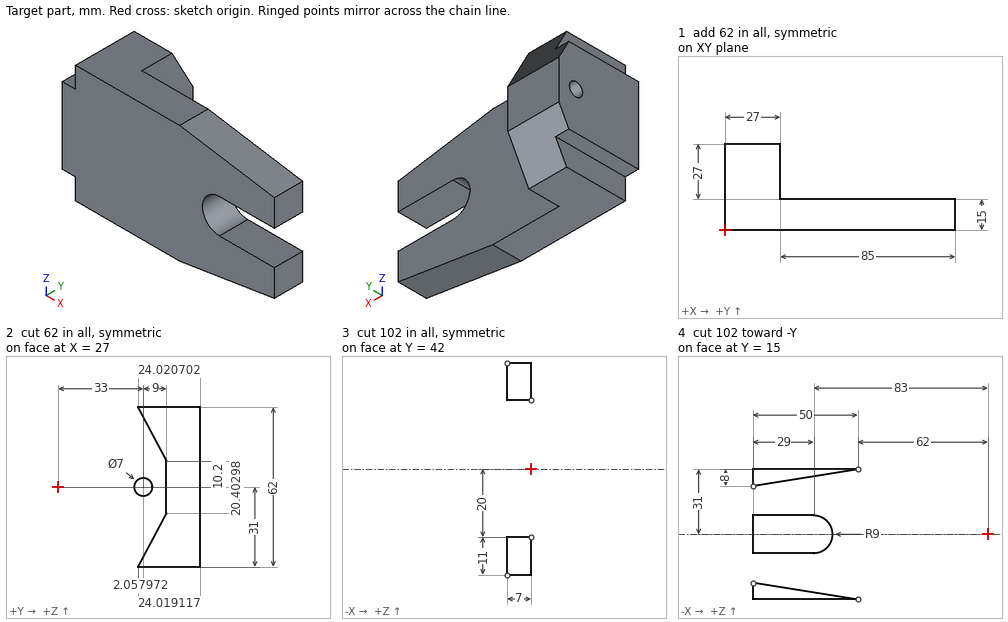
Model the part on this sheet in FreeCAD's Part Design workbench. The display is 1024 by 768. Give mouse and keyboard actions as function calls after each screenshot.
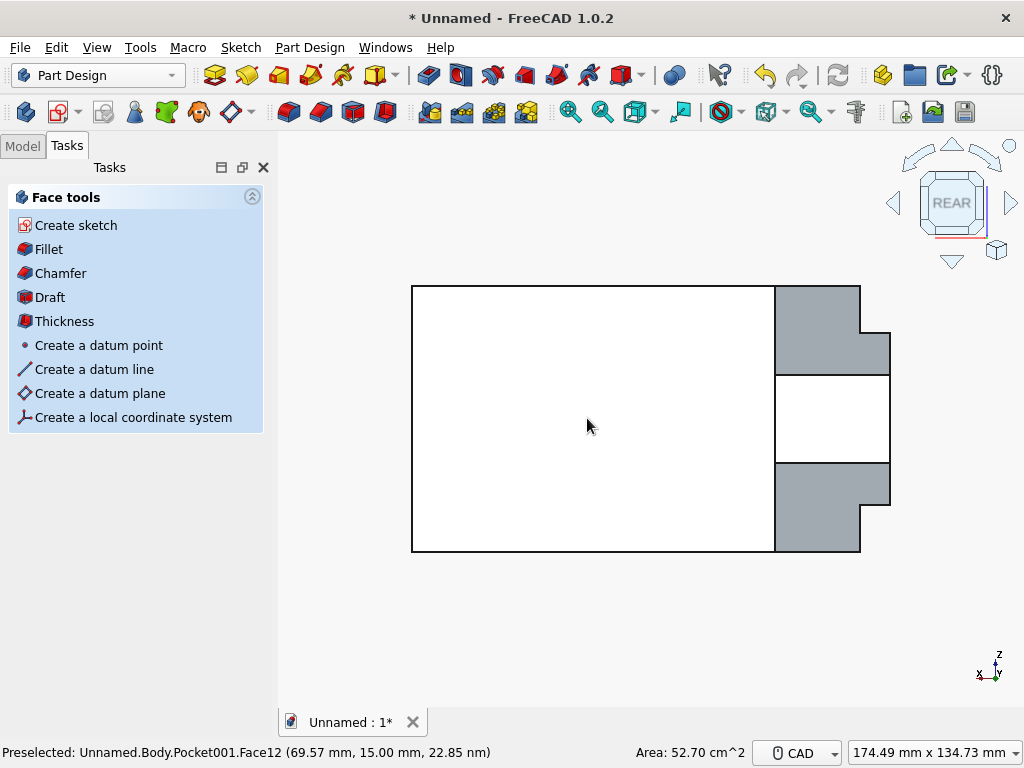
click(58, 112)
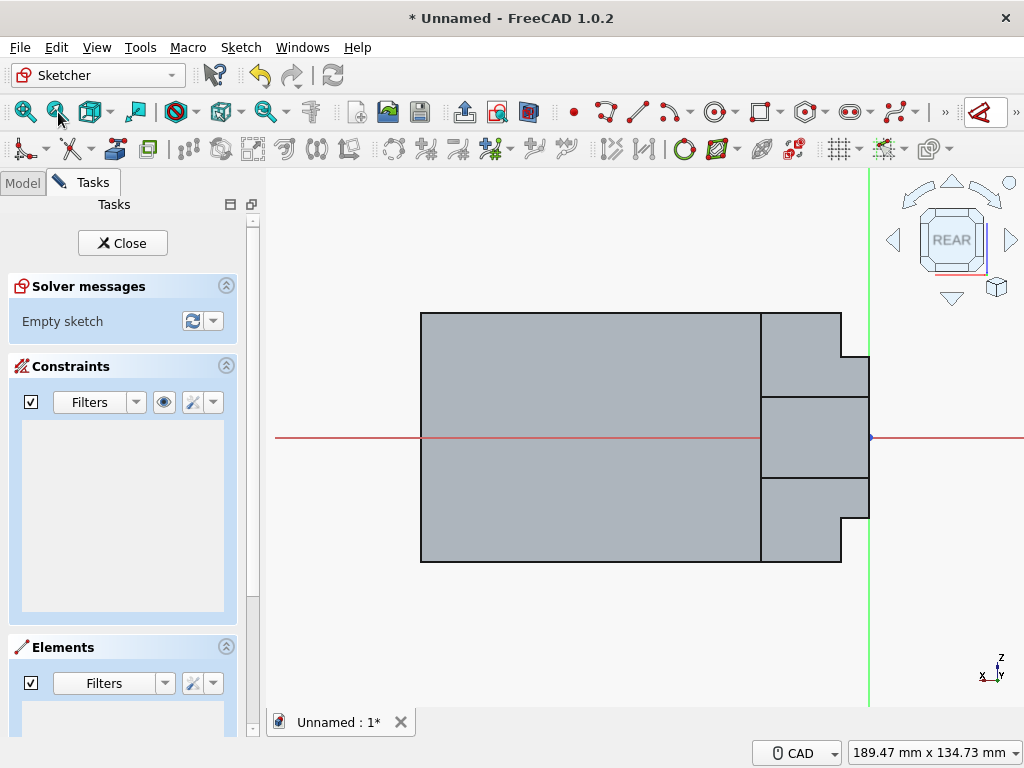
click(530, 112)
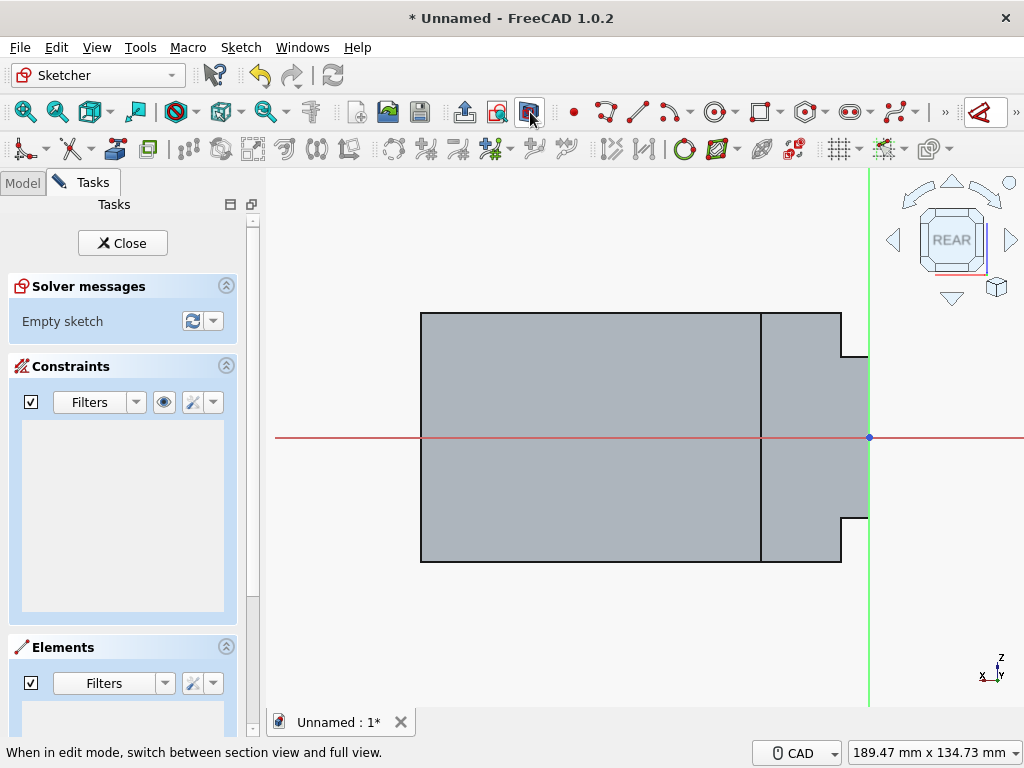
scroll(294, 437, down, 1)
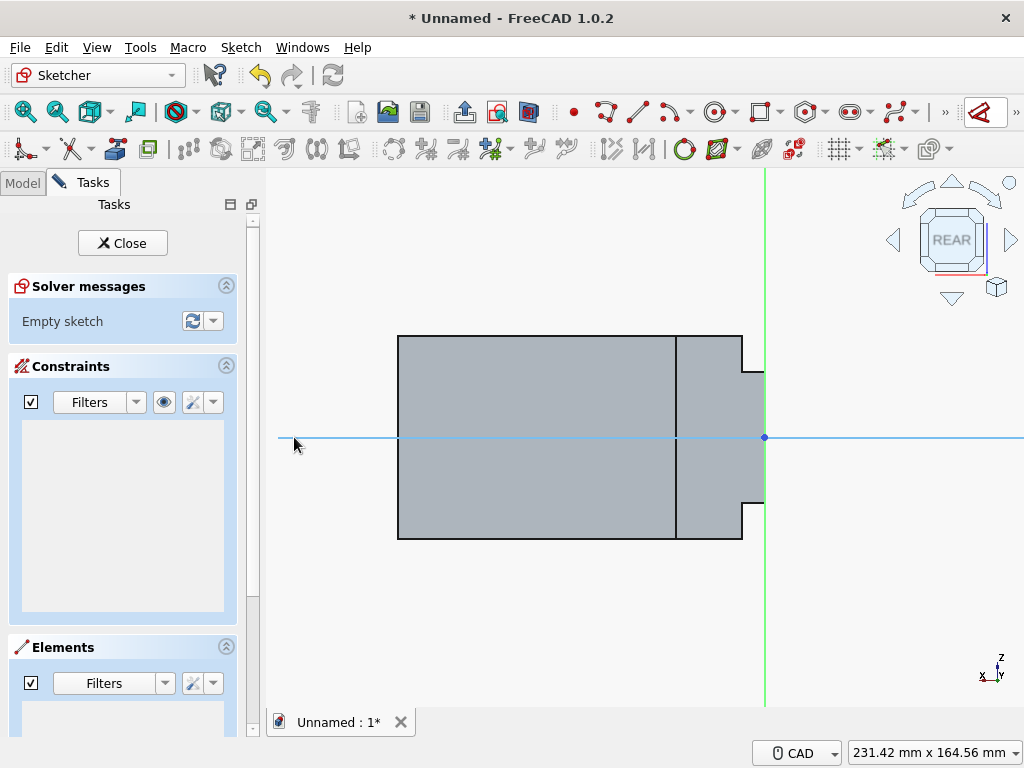
click(606, 112)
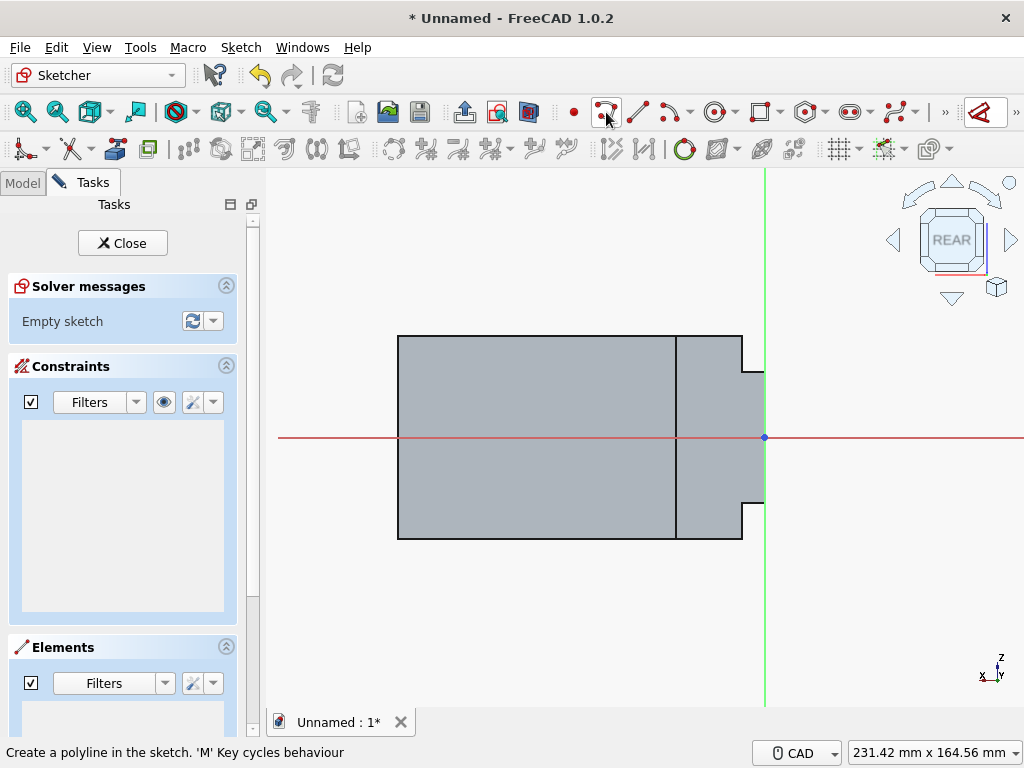
click(562, 336)
click(398, 336)
click(398, 362)
click(562, 337)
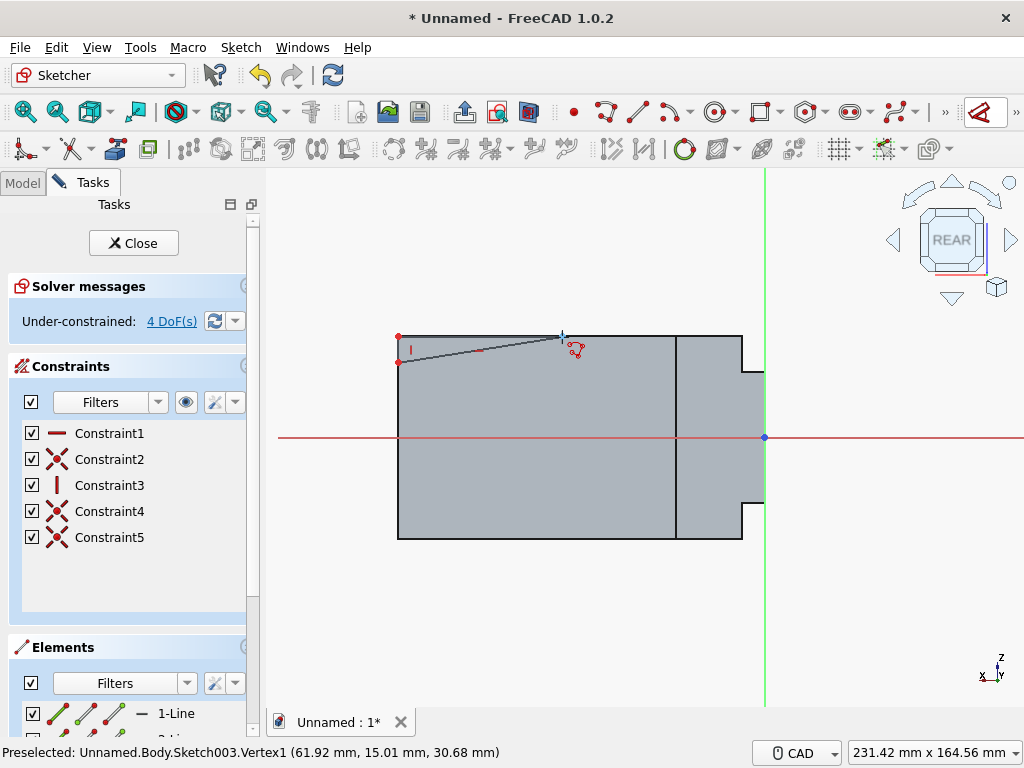
click(562, 539)
click(398, 513)
click(398, 539)
click(562, 540)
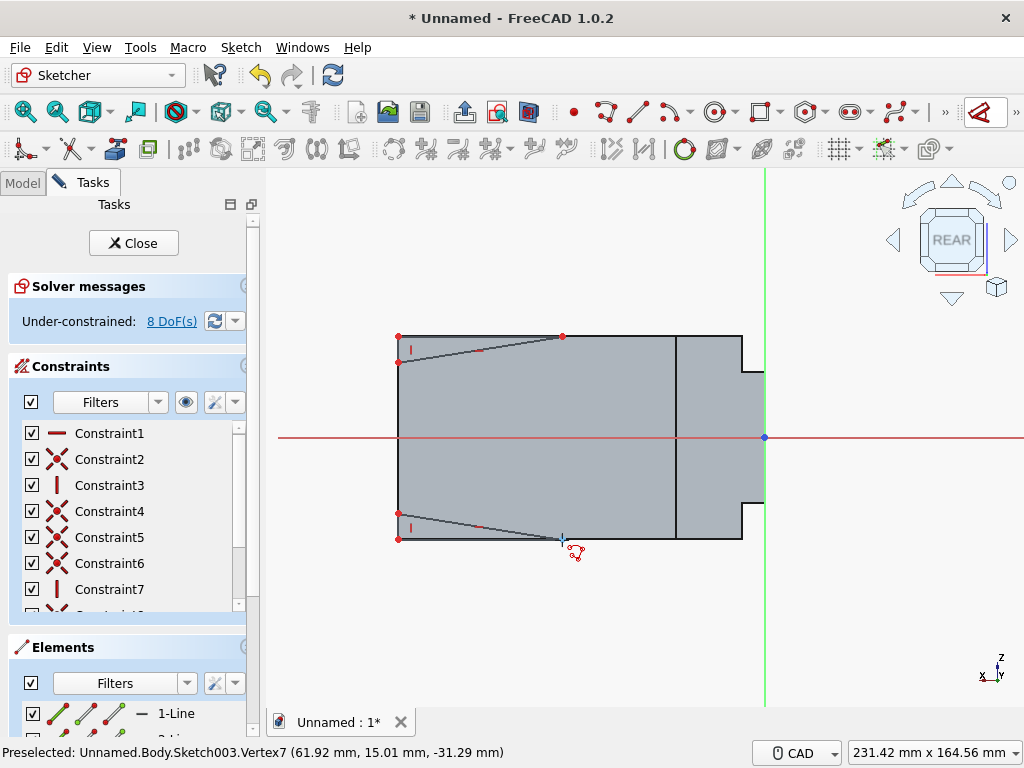
click(493, 408)
click(398, 408)
click(398, 467)
click(493, 467)
right_click(493, 467)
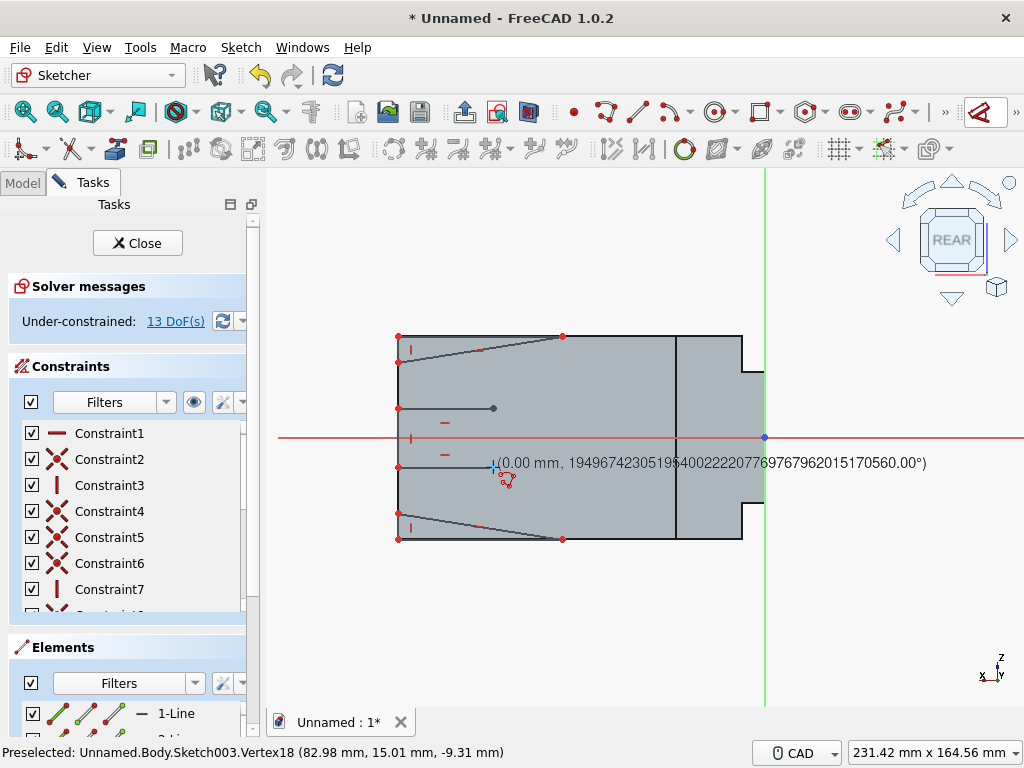
click(692, 112)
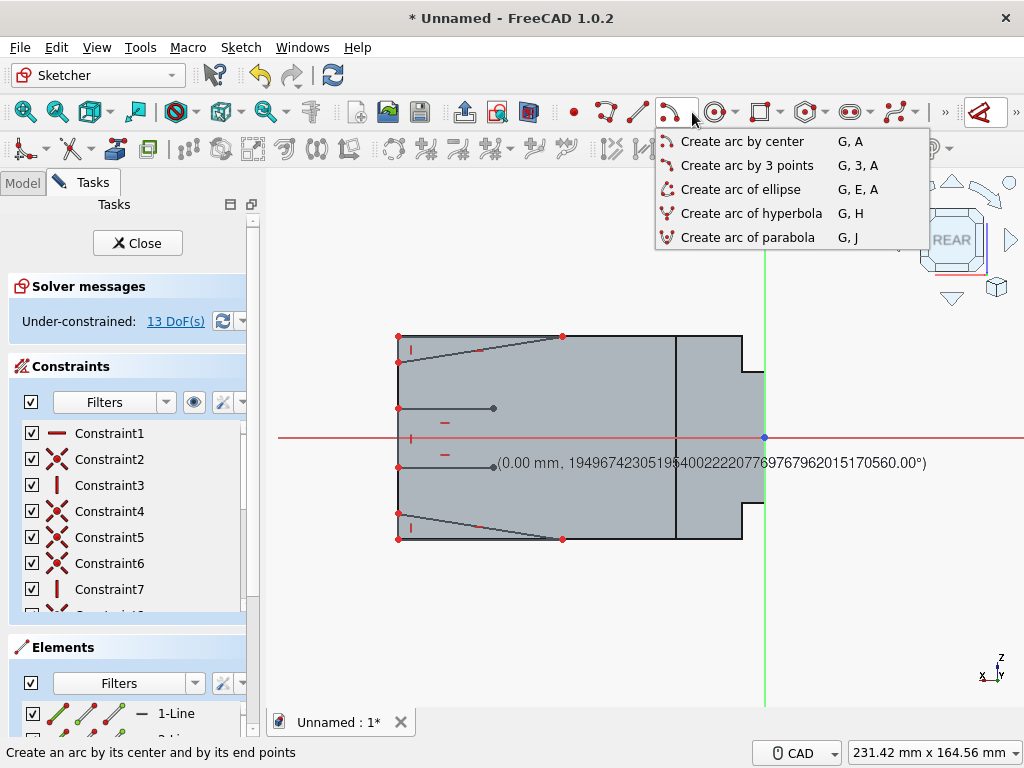
click(792, 165)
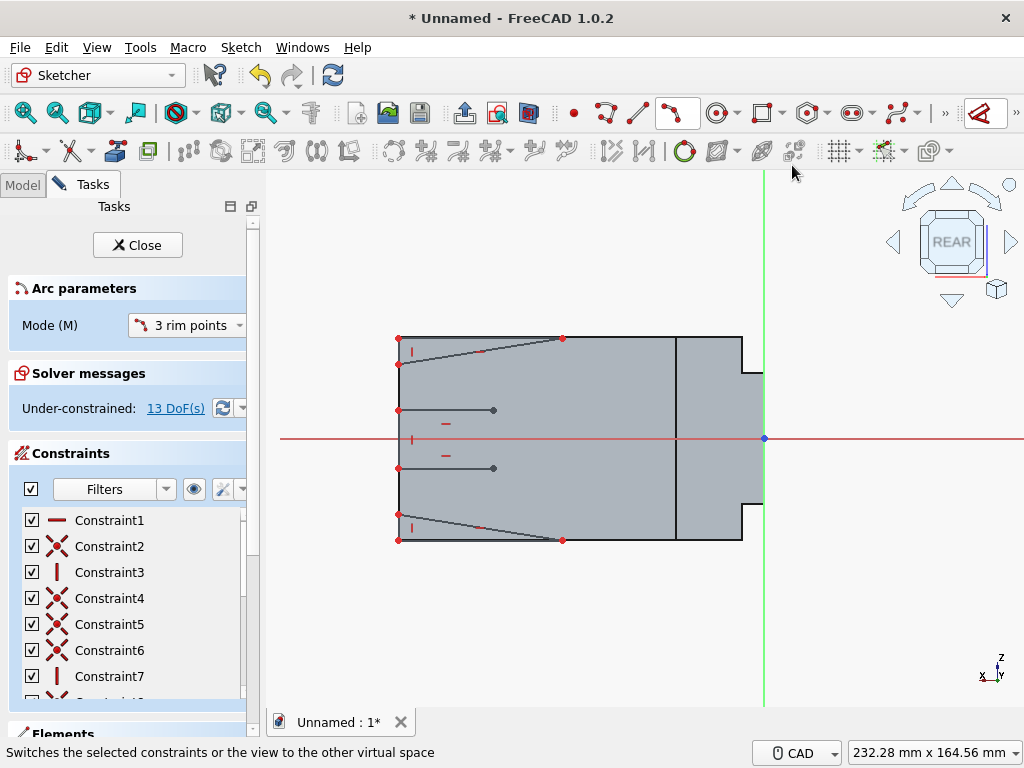
click(494, 469)
click(494, 410)
click(517, 456)
key(Escape)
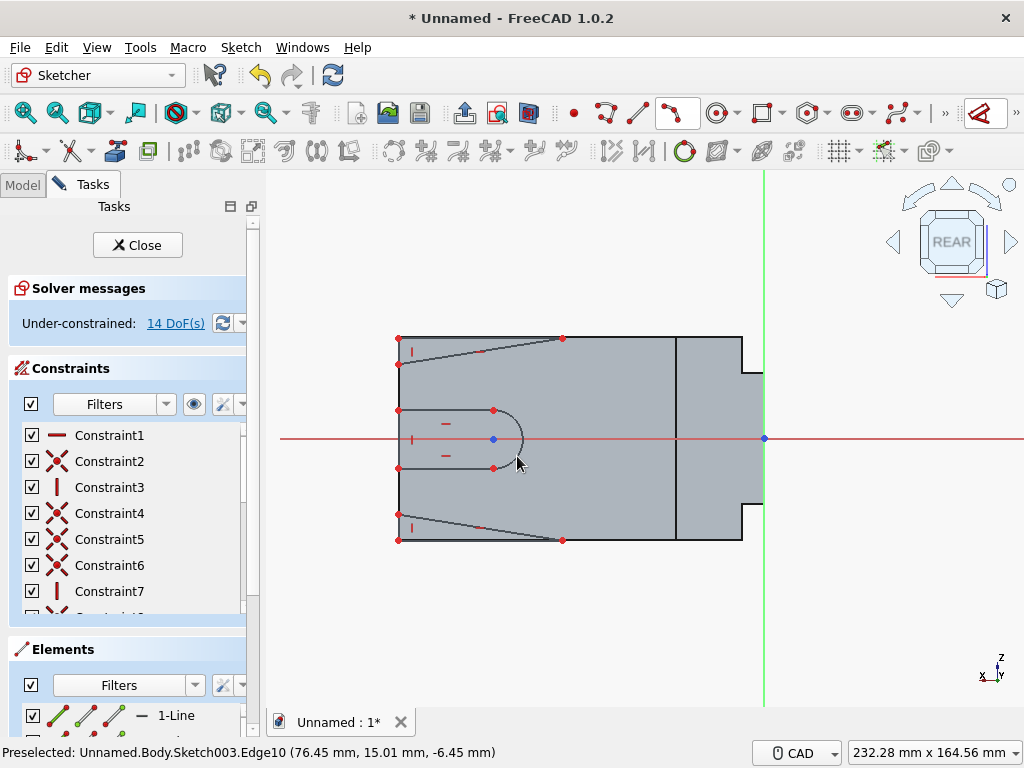
click(465, 410)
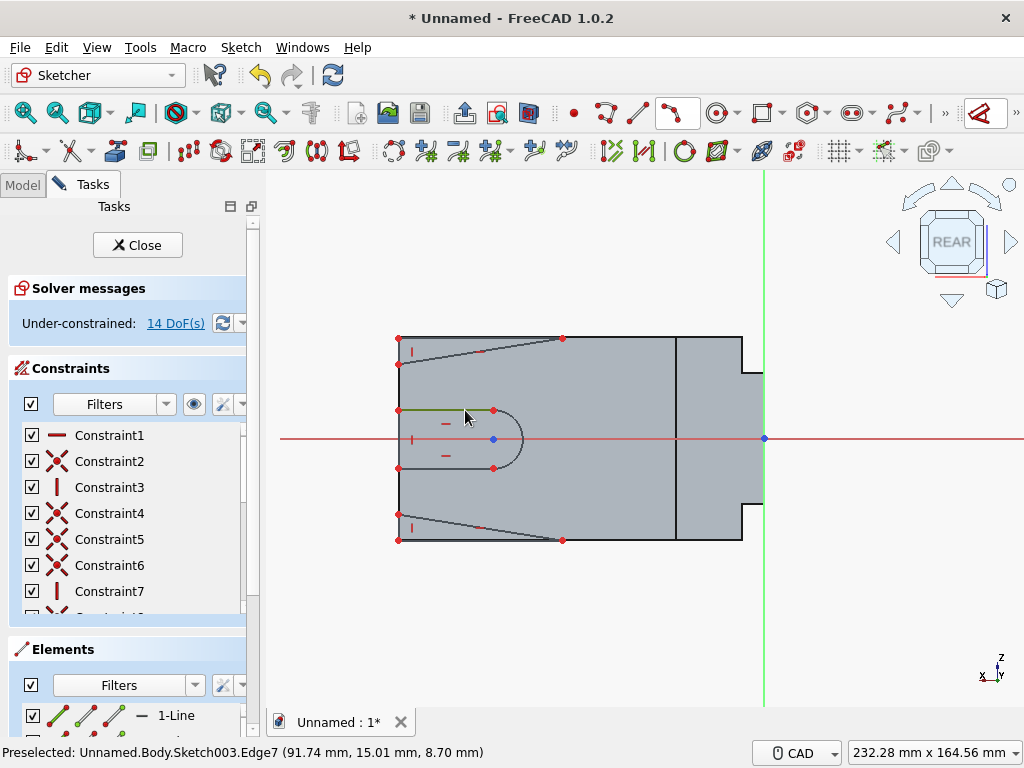
click(517, 457)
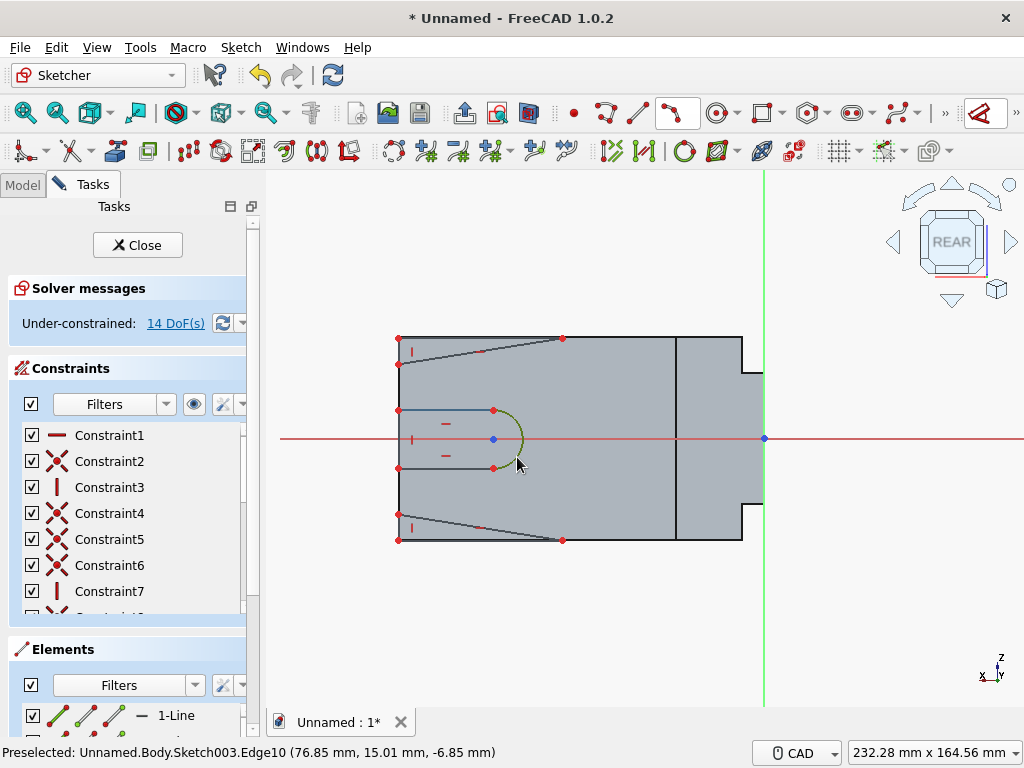
key(t)